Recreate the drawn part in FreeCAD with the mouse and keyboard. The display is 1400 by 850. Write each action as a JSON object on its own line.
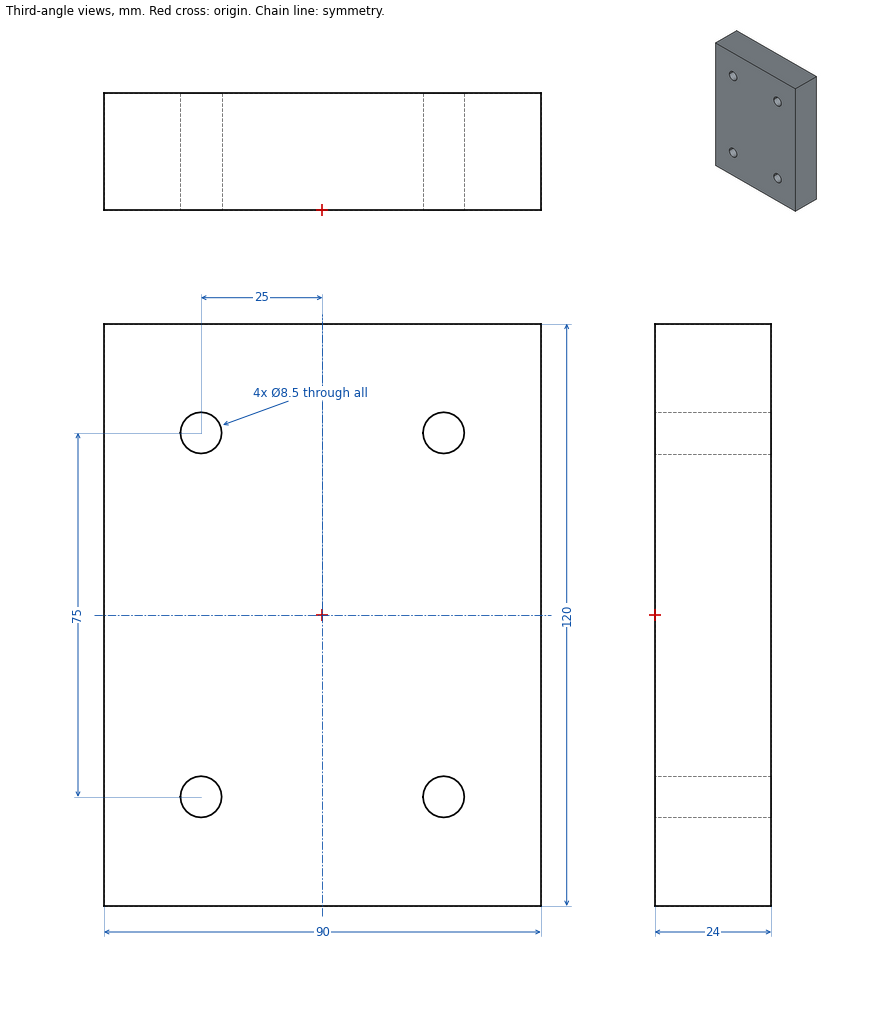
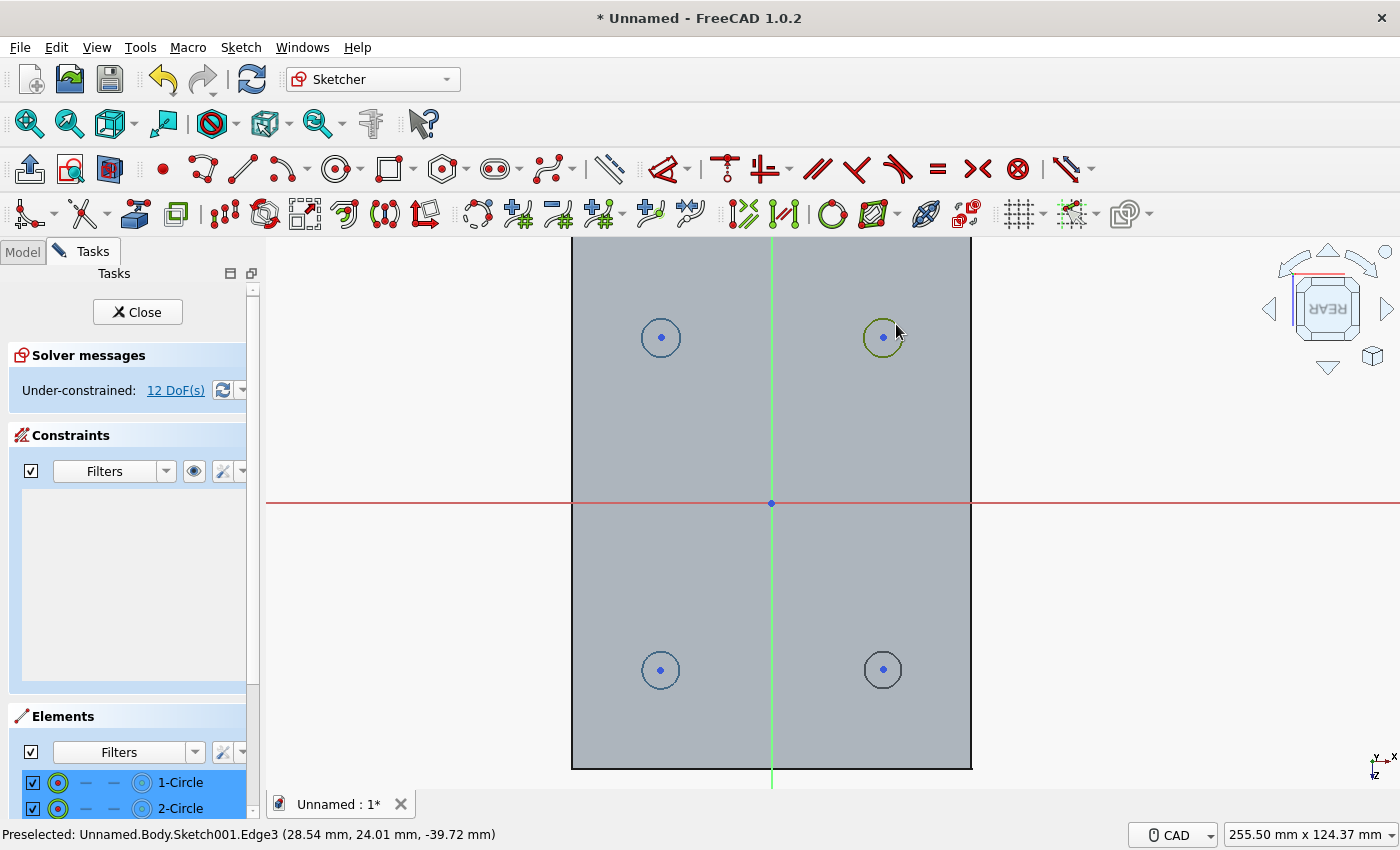
{"action": "left_click", "coordinate": [896, 657]}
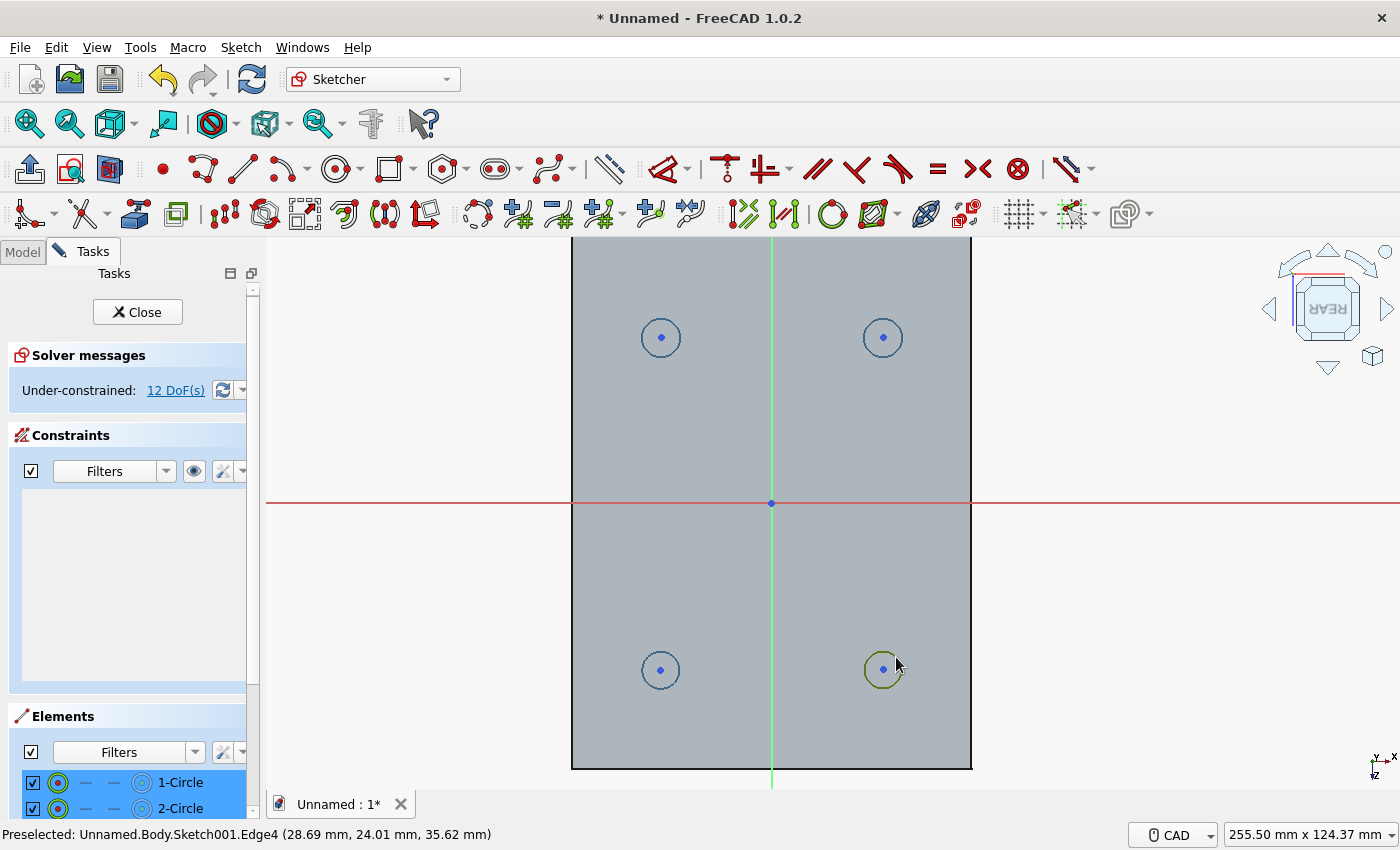
{"action": "key", "text": "e"}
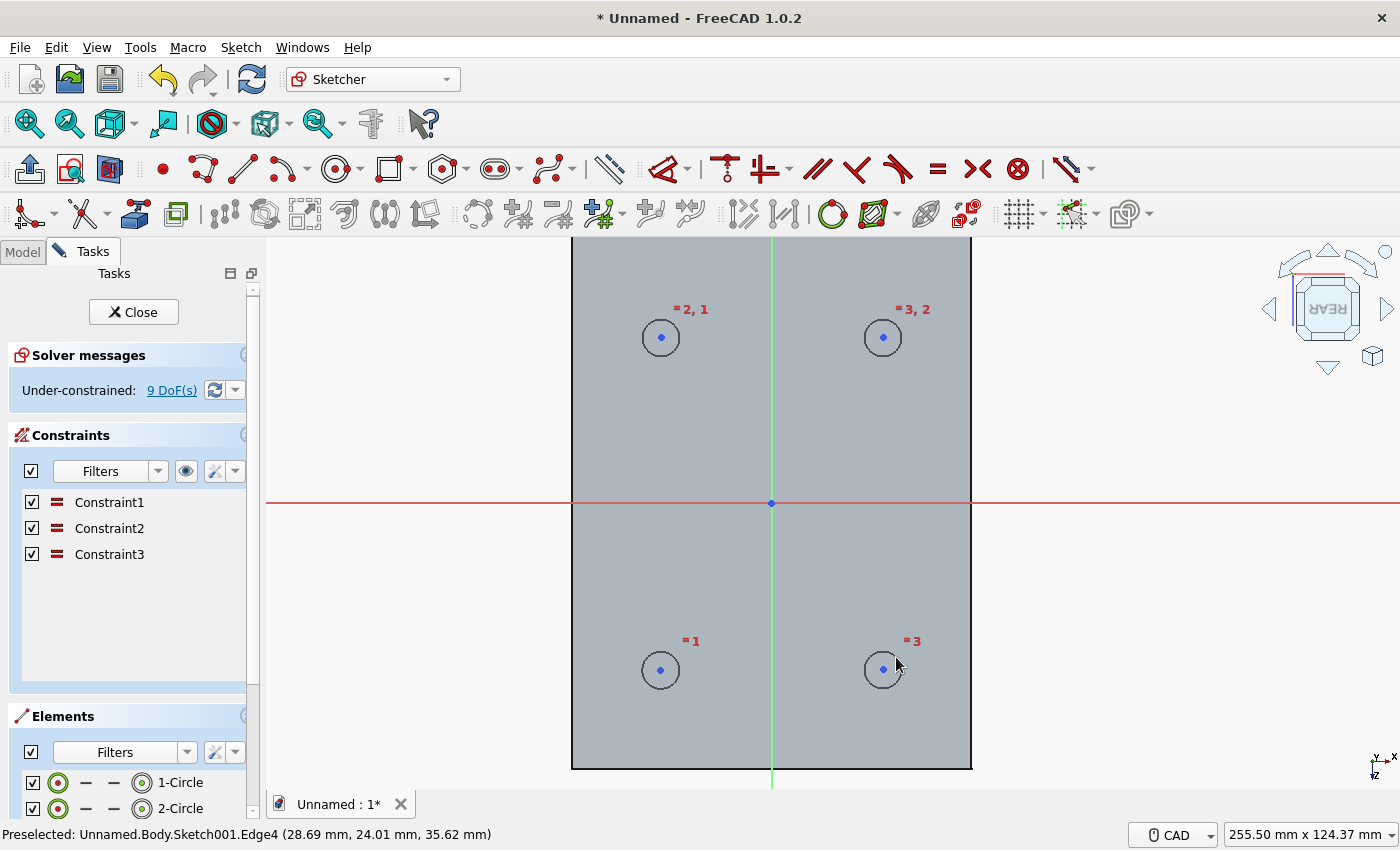
{"action": "left_click", "coordinate": [661, 670]}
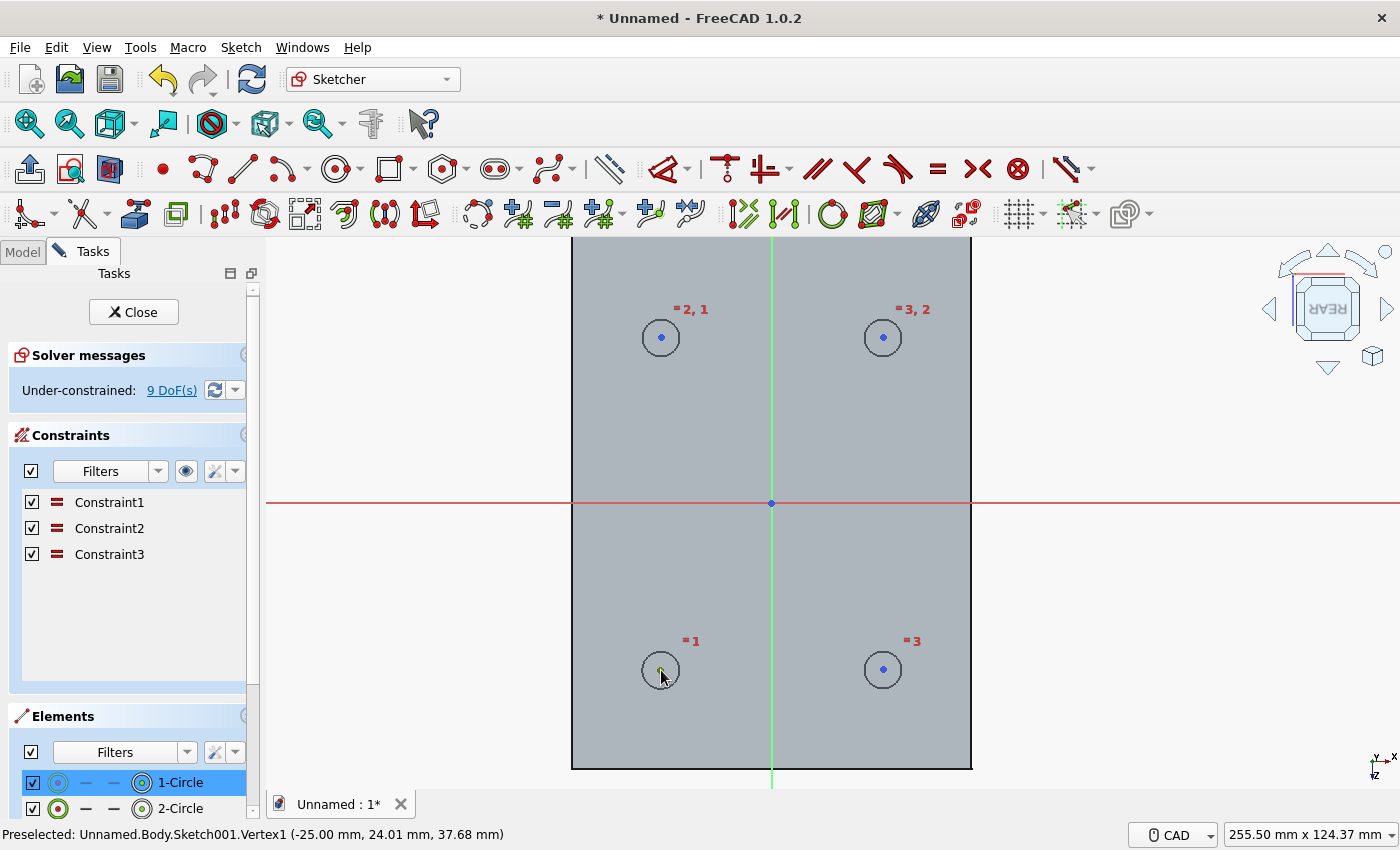
{"action": "left_click", "coordinate": [661, 338]}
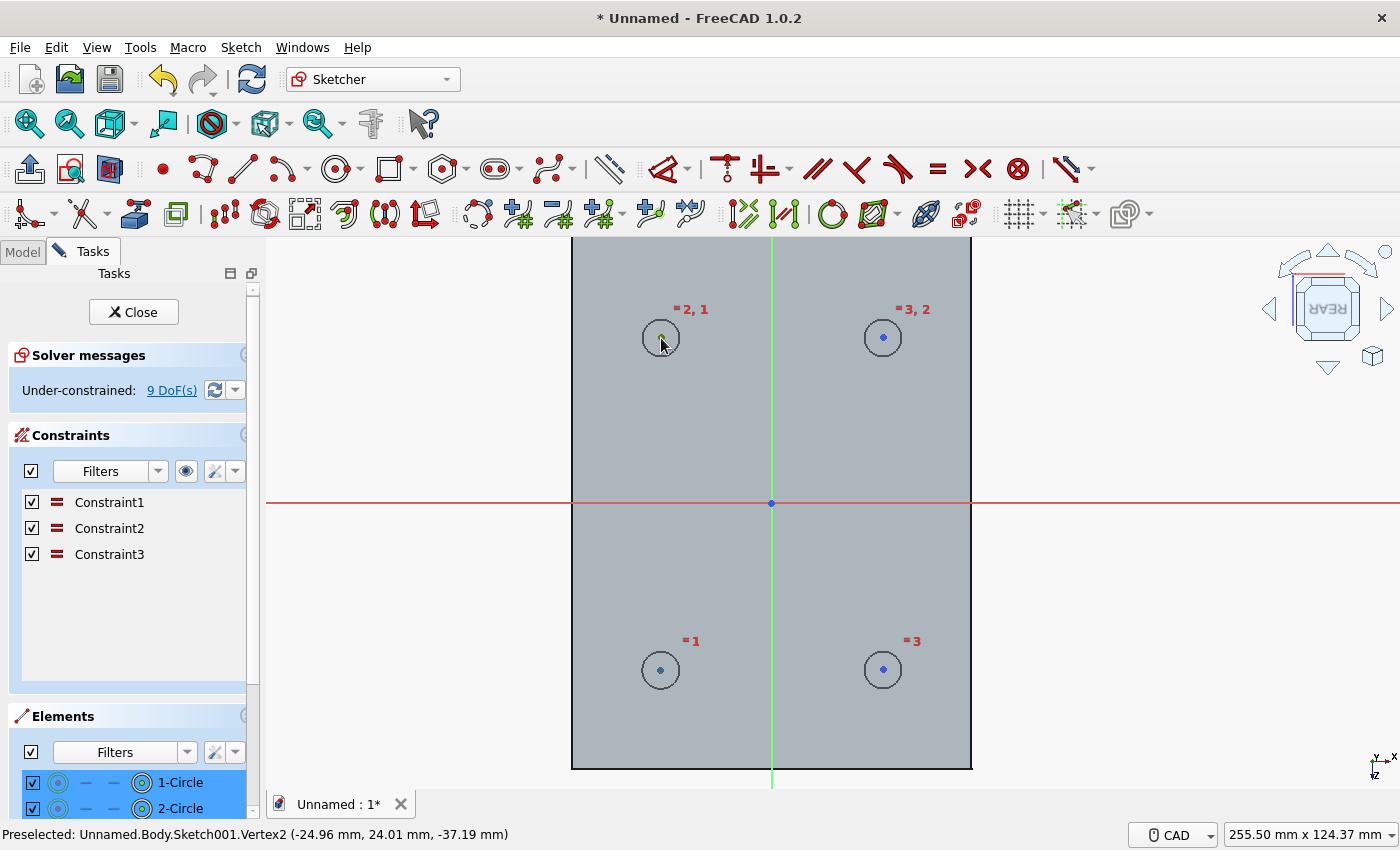
{"action": "left_click", "coordinate": [361, 503]}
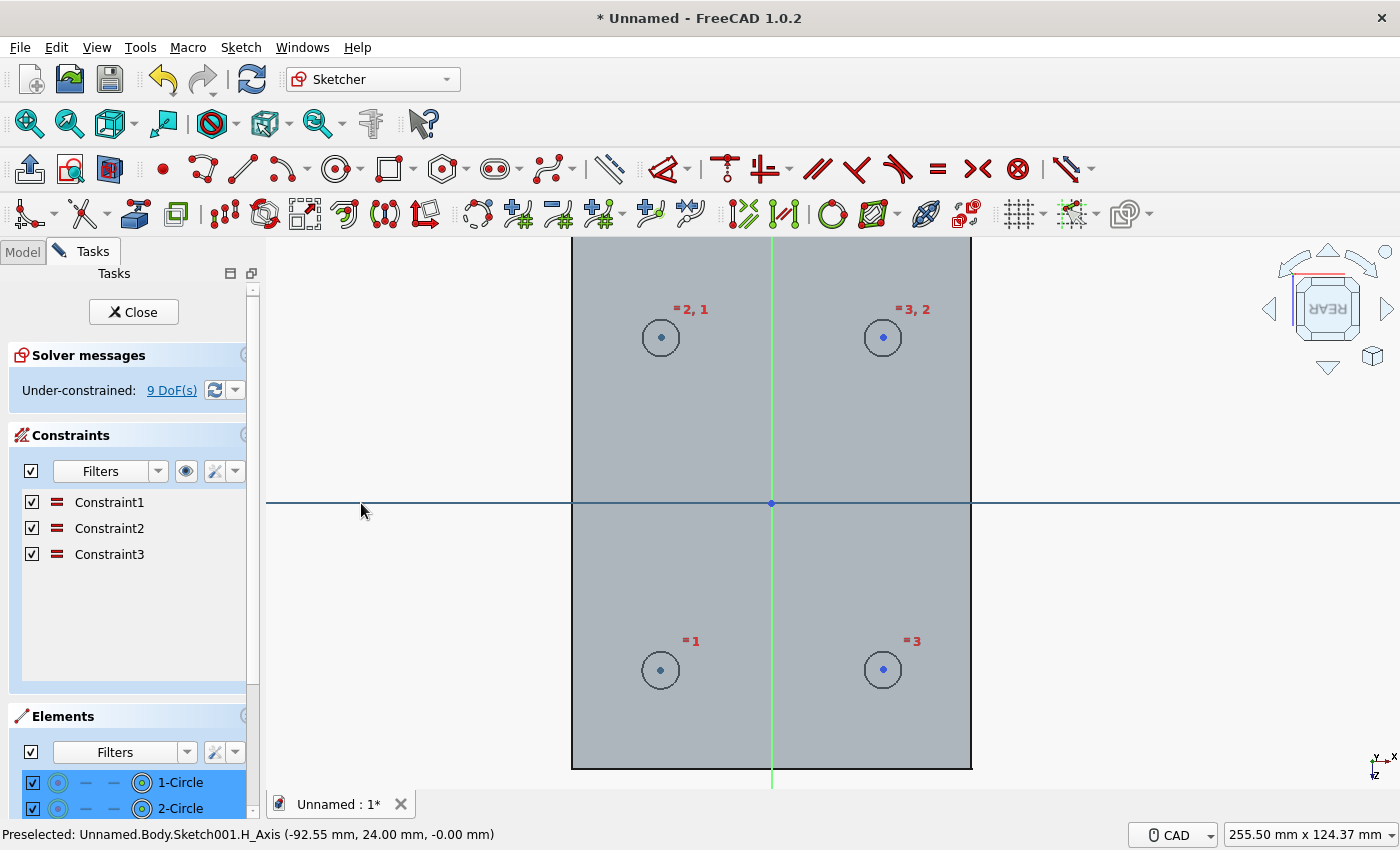
{"action": "key", "text": "s"}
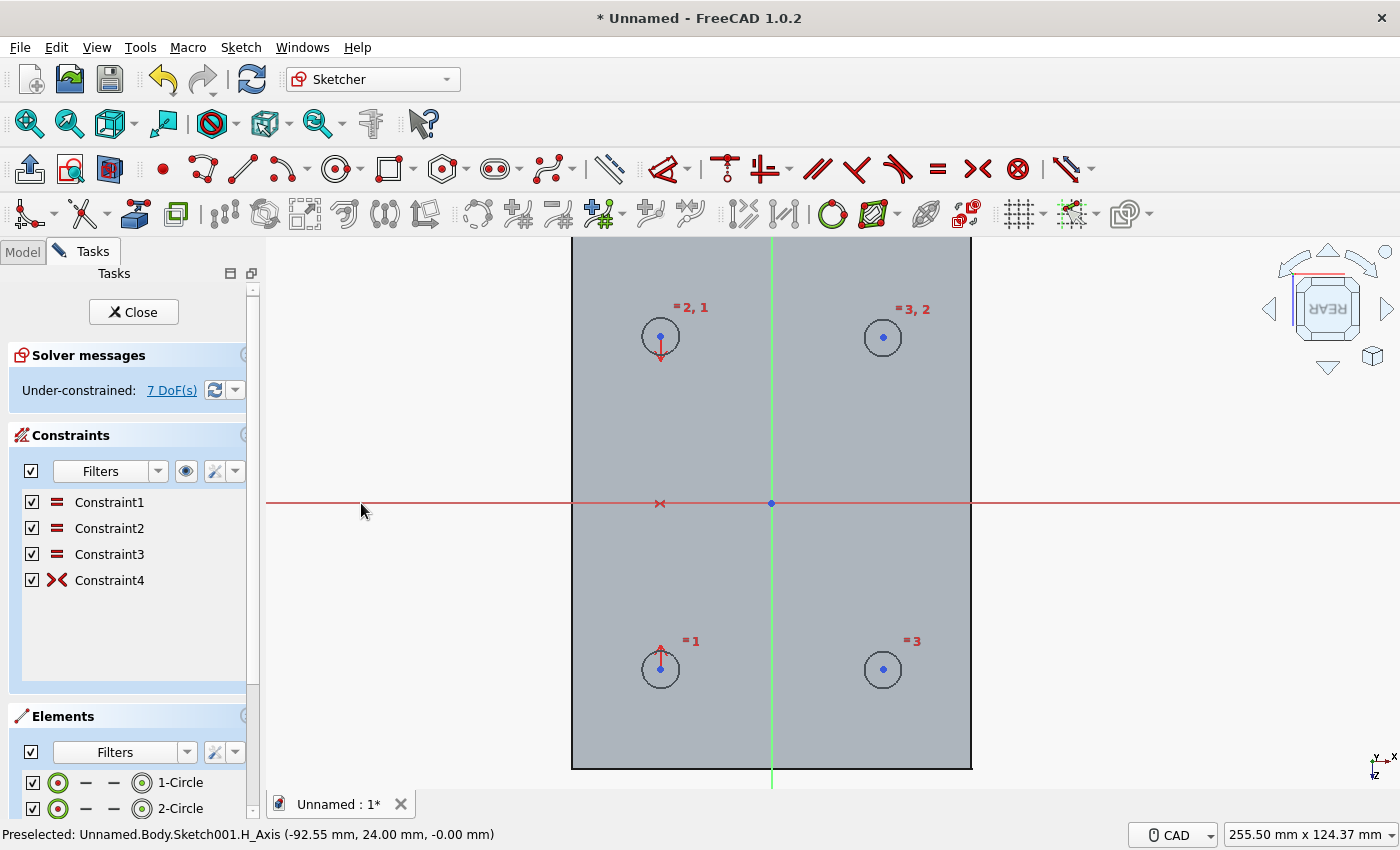
{"action": "left_click", "coordinate": [661, 336]}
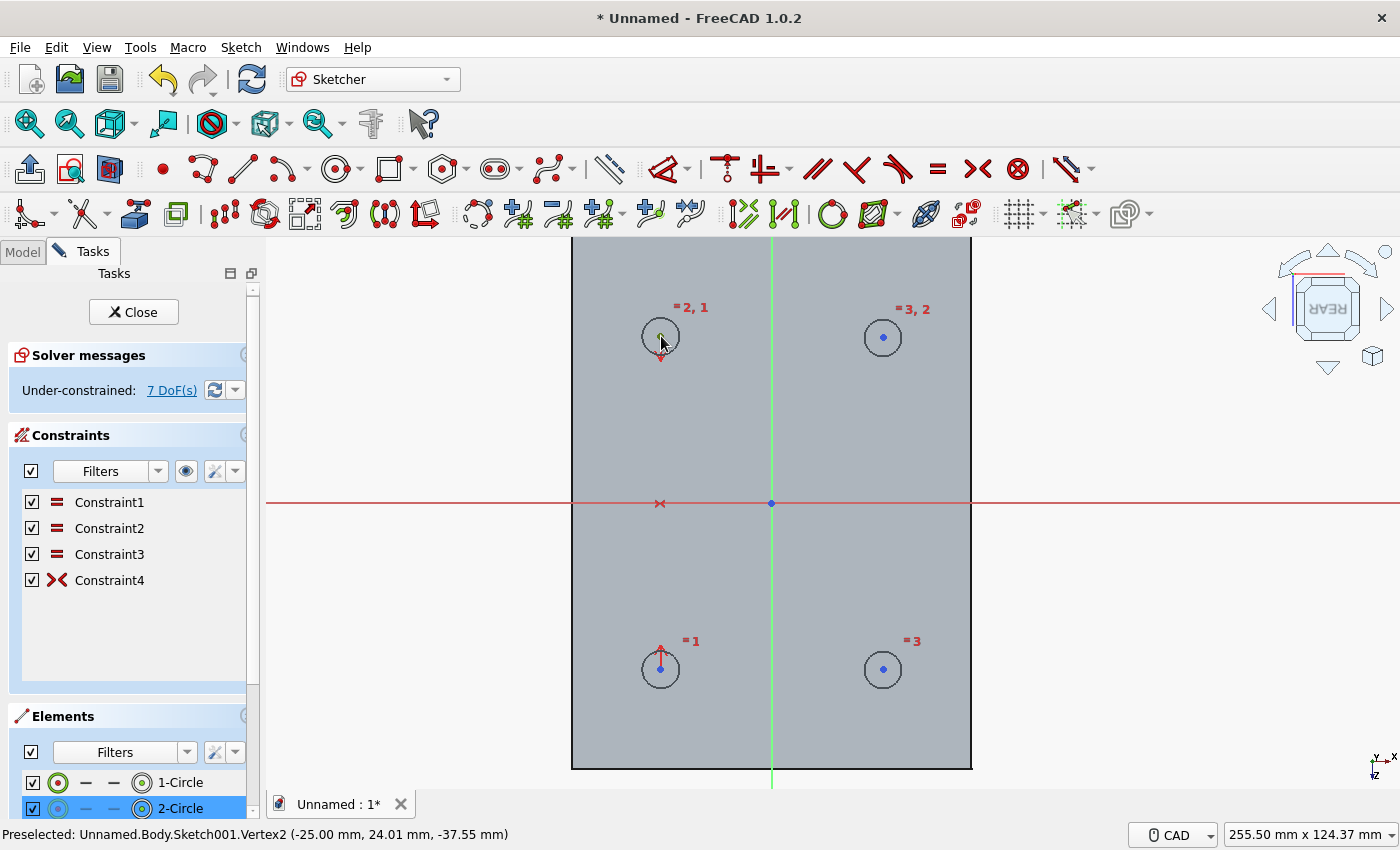
{"action": "left_click", "coordinate": [883, 338]}